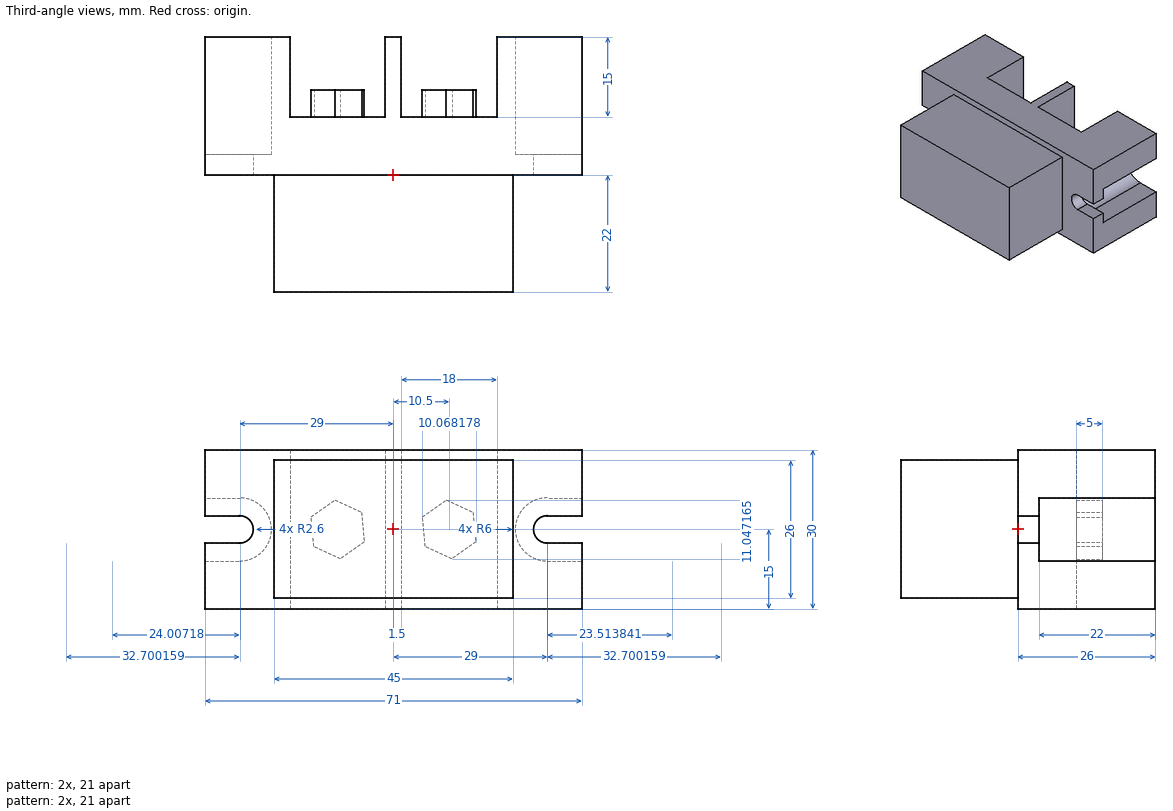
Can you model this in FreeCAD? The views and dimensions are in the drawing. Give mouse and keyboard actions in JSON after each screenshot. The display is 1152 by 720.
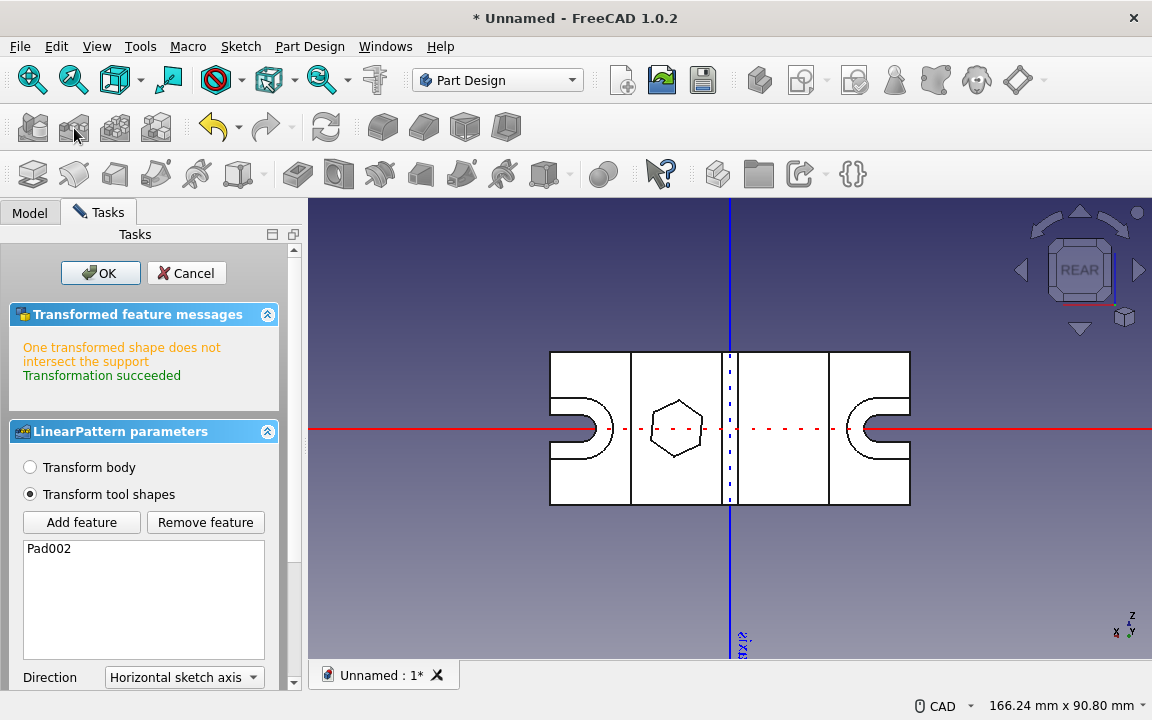
{"action": "left_click", "coordinate": [185, 678]}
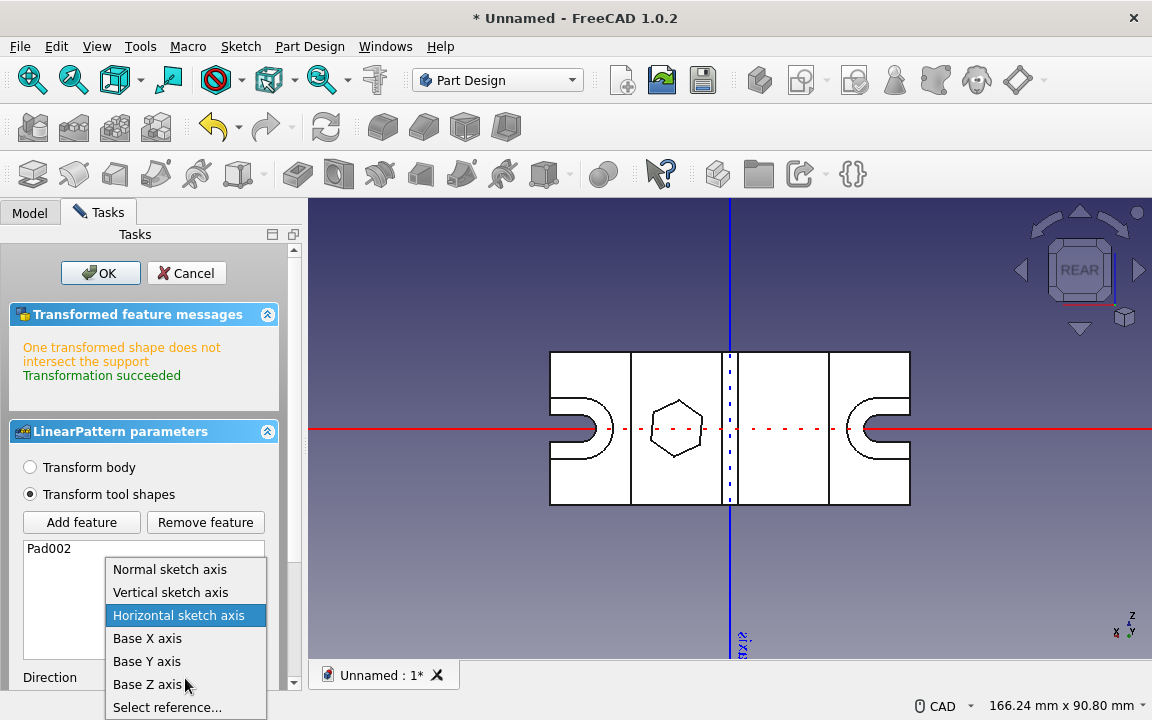
{"action": "left_click", "coordinate": [184, 638]}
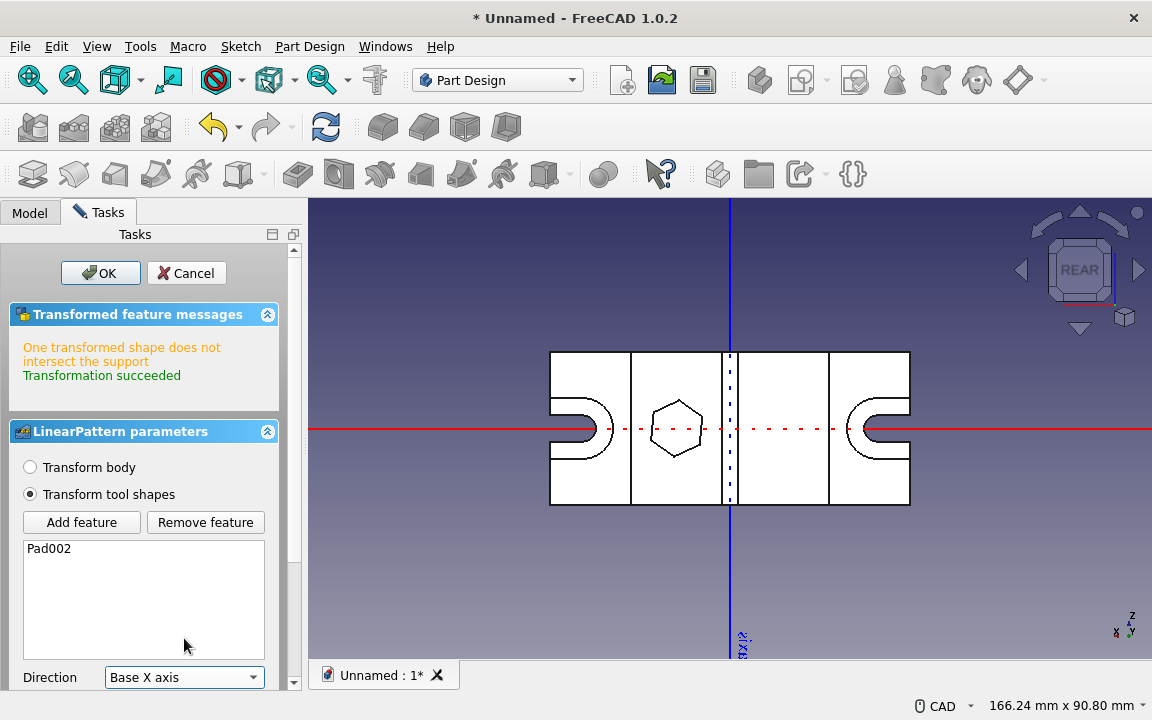
{"action": "scroll", "coordinate": [294, 467], "scroll_direction": "down", "scroll_amount": 2}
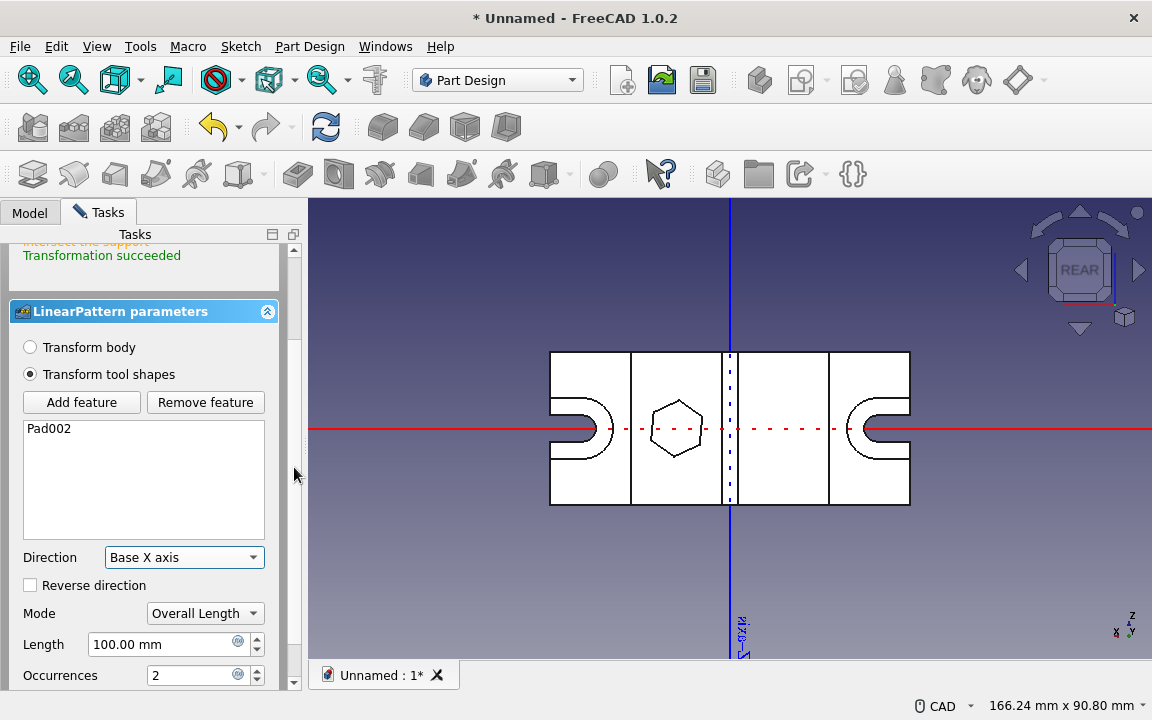
{"action": "left_click", "coordinate": [206, 614]}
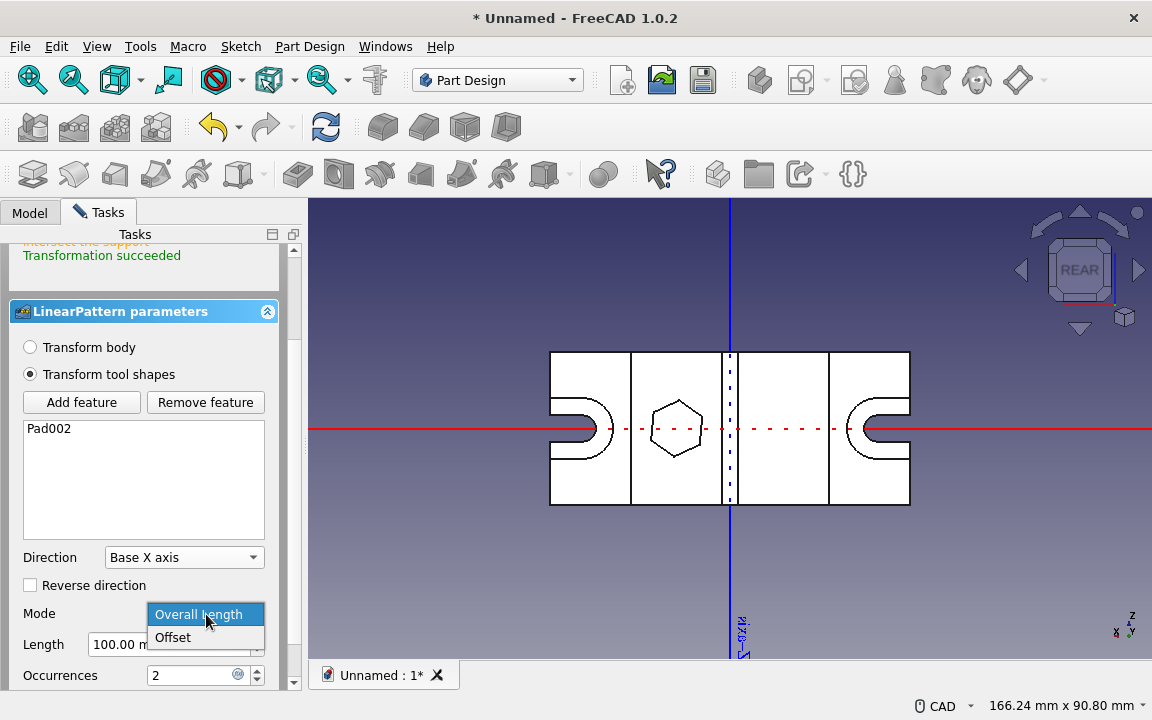
{"action": "left_click", "coordinate": [204, 638]}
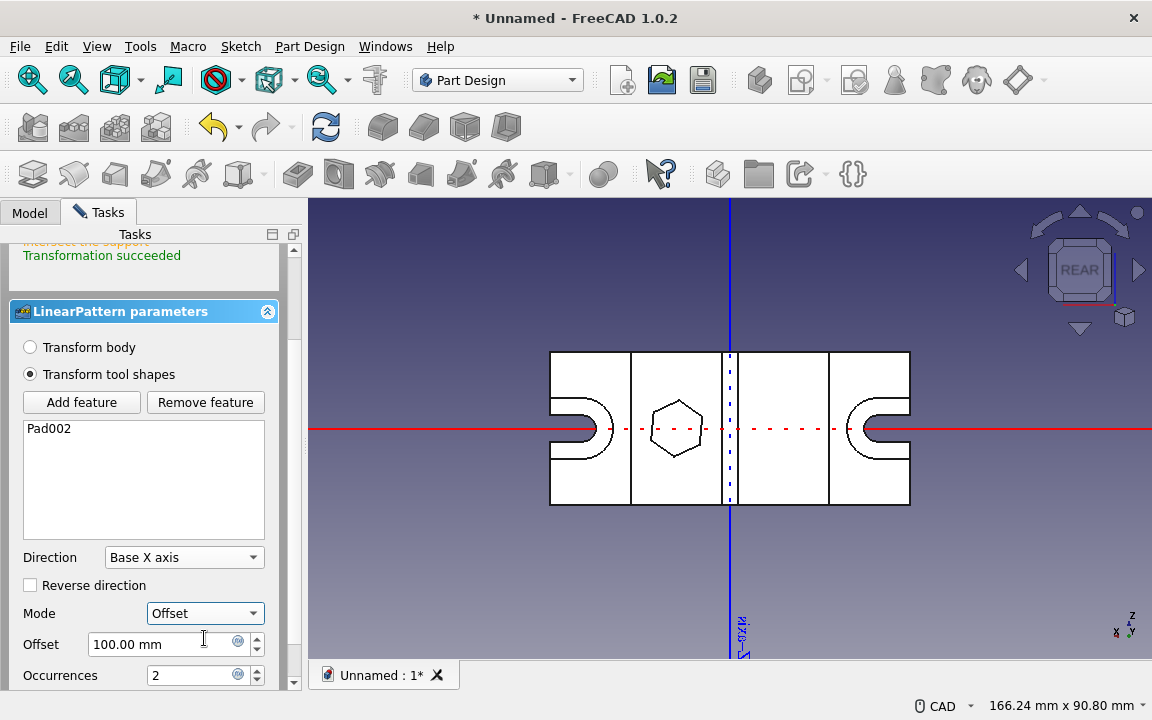
{"action": "triple_click", "coordinate": [170, 644]}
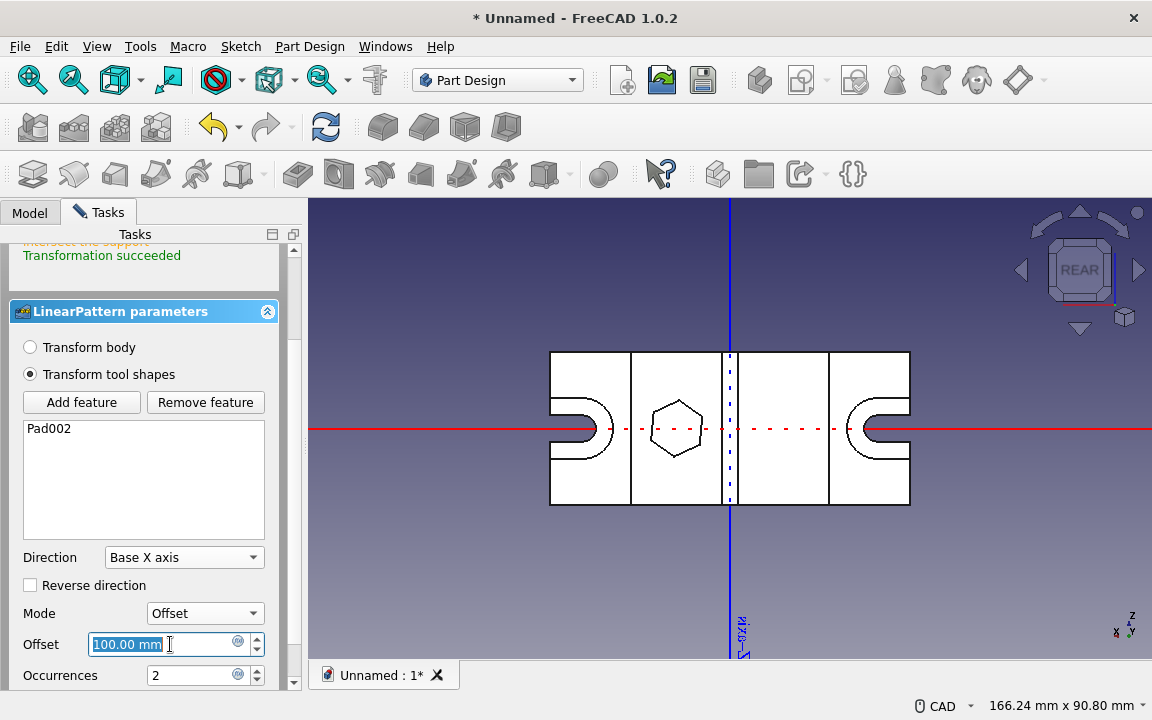
{"action": "type", "text": "21"}
{"action": "key", "text": "Tab"}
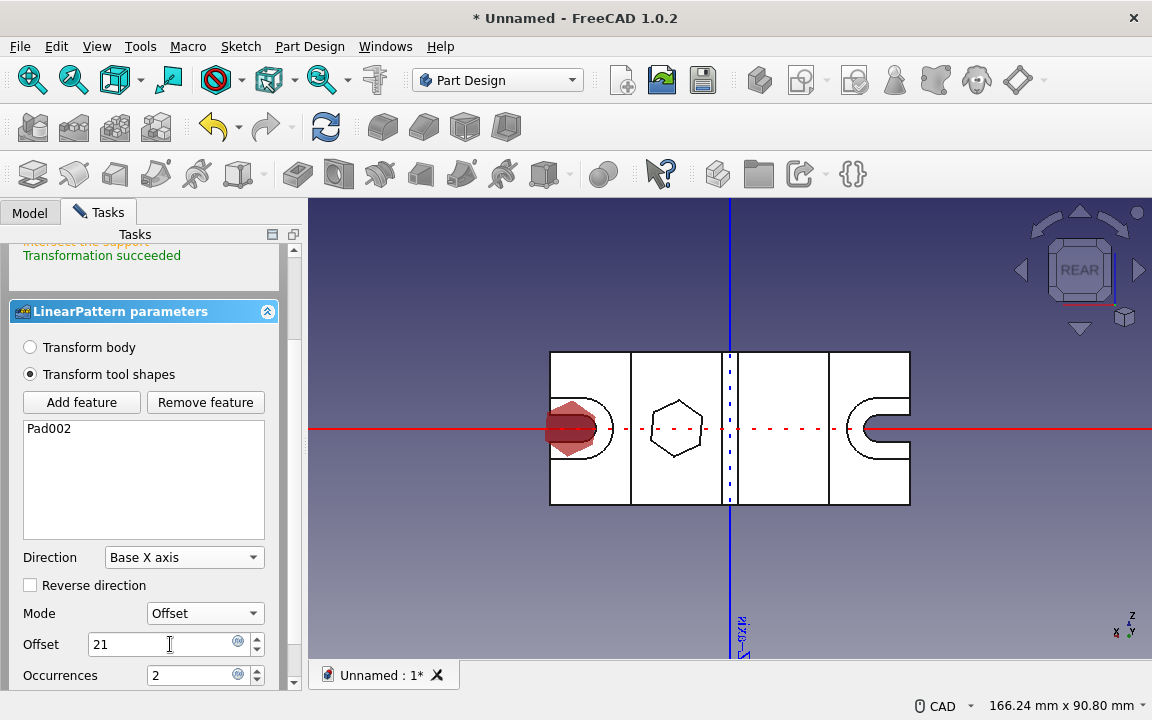
{"action": "triple_click", "coordinate": [199, 676]}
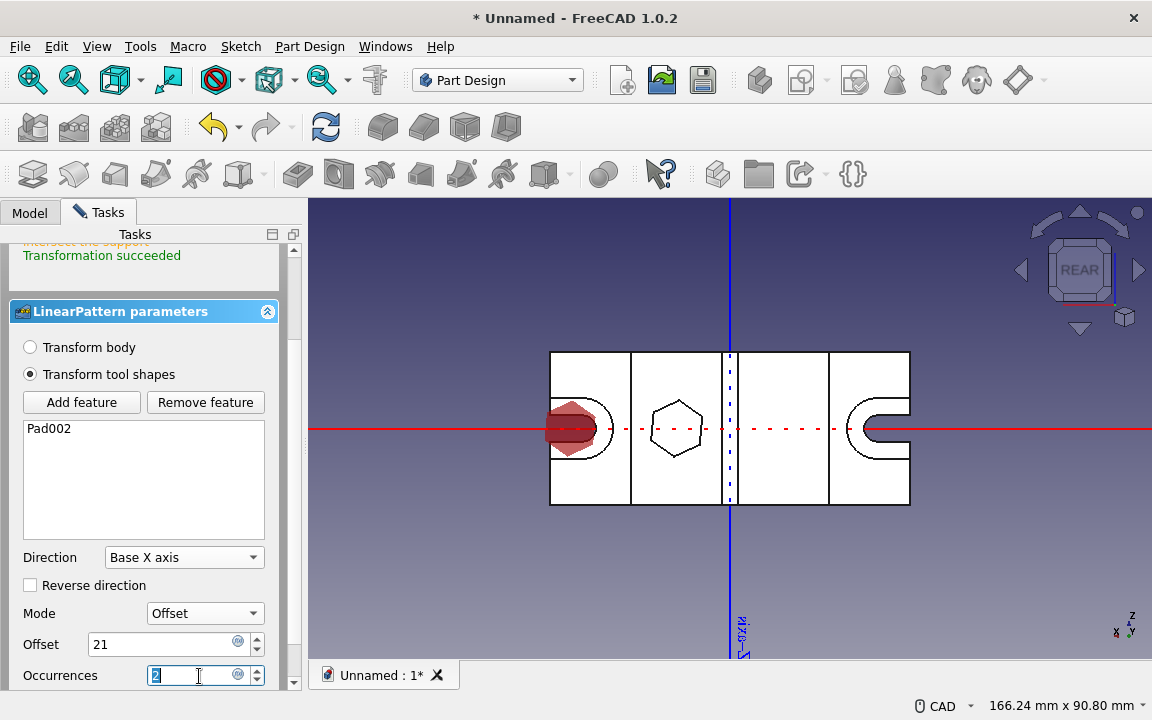
{"action": "type", "text": "2"}
{"action": "key", "text": "Tab"}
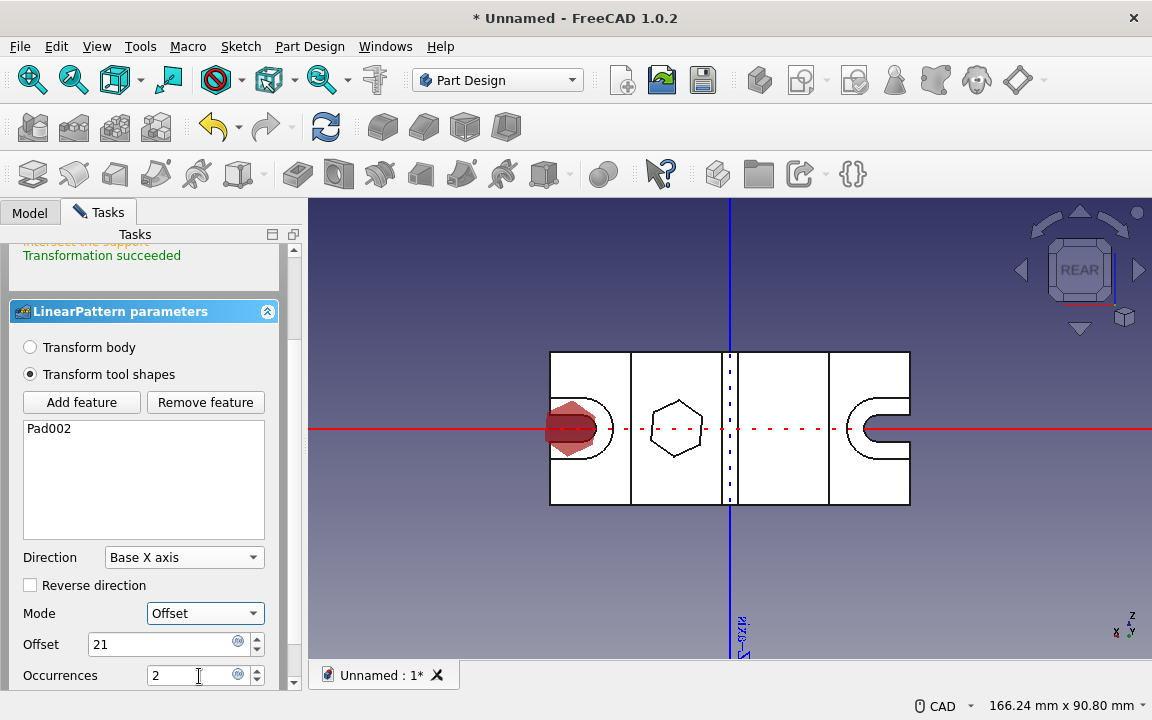
{"action": "left_click", "coordinate": [31, 585]}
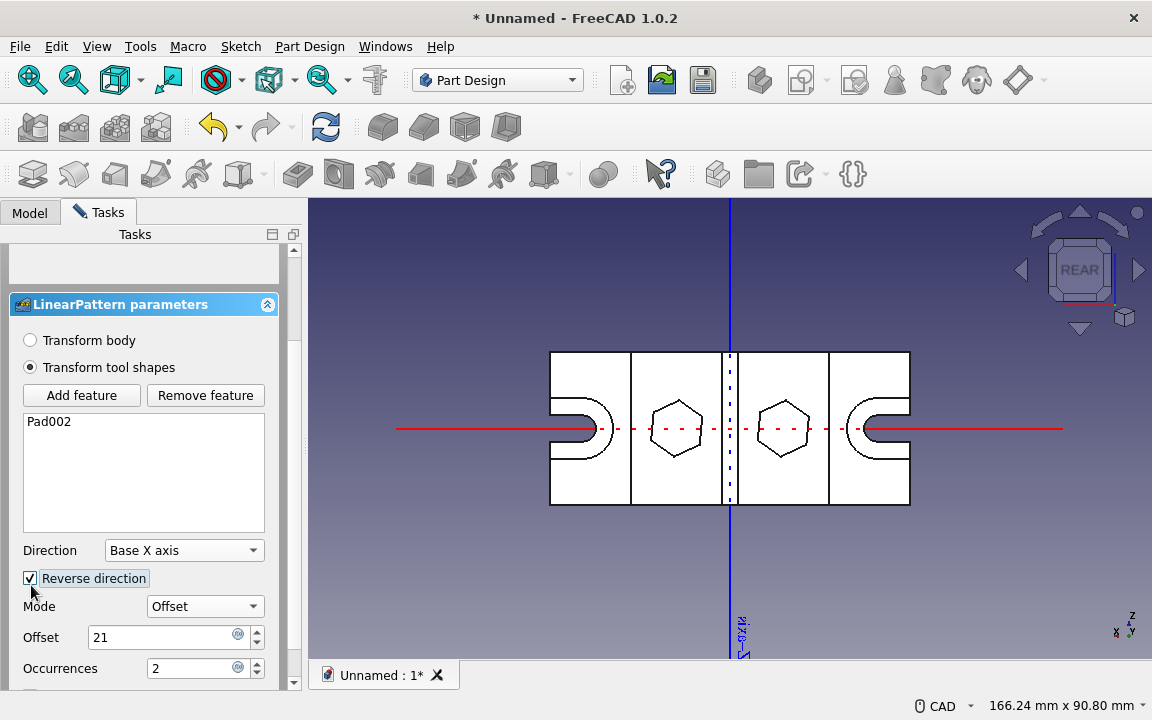
{"action": "scroll", "coordinate": [294, 467], "scroll_direction": "up", "scroll_amount": 3}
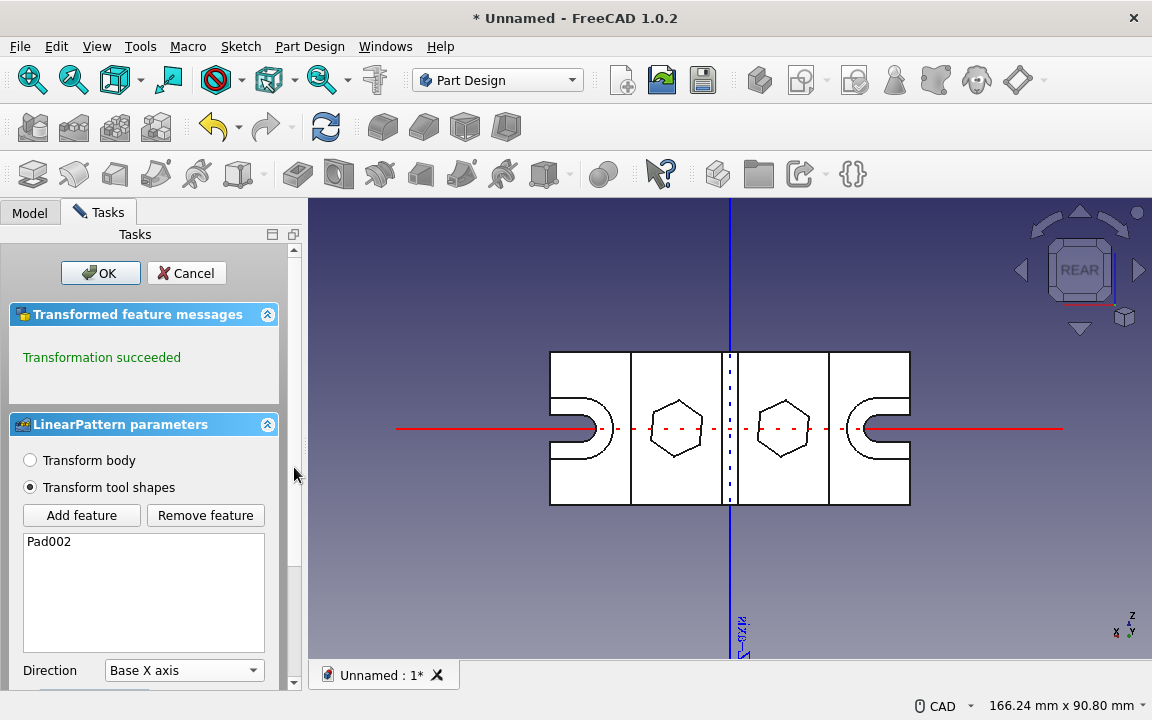
{"action": "left_click", "coordinate": [101, 273]}